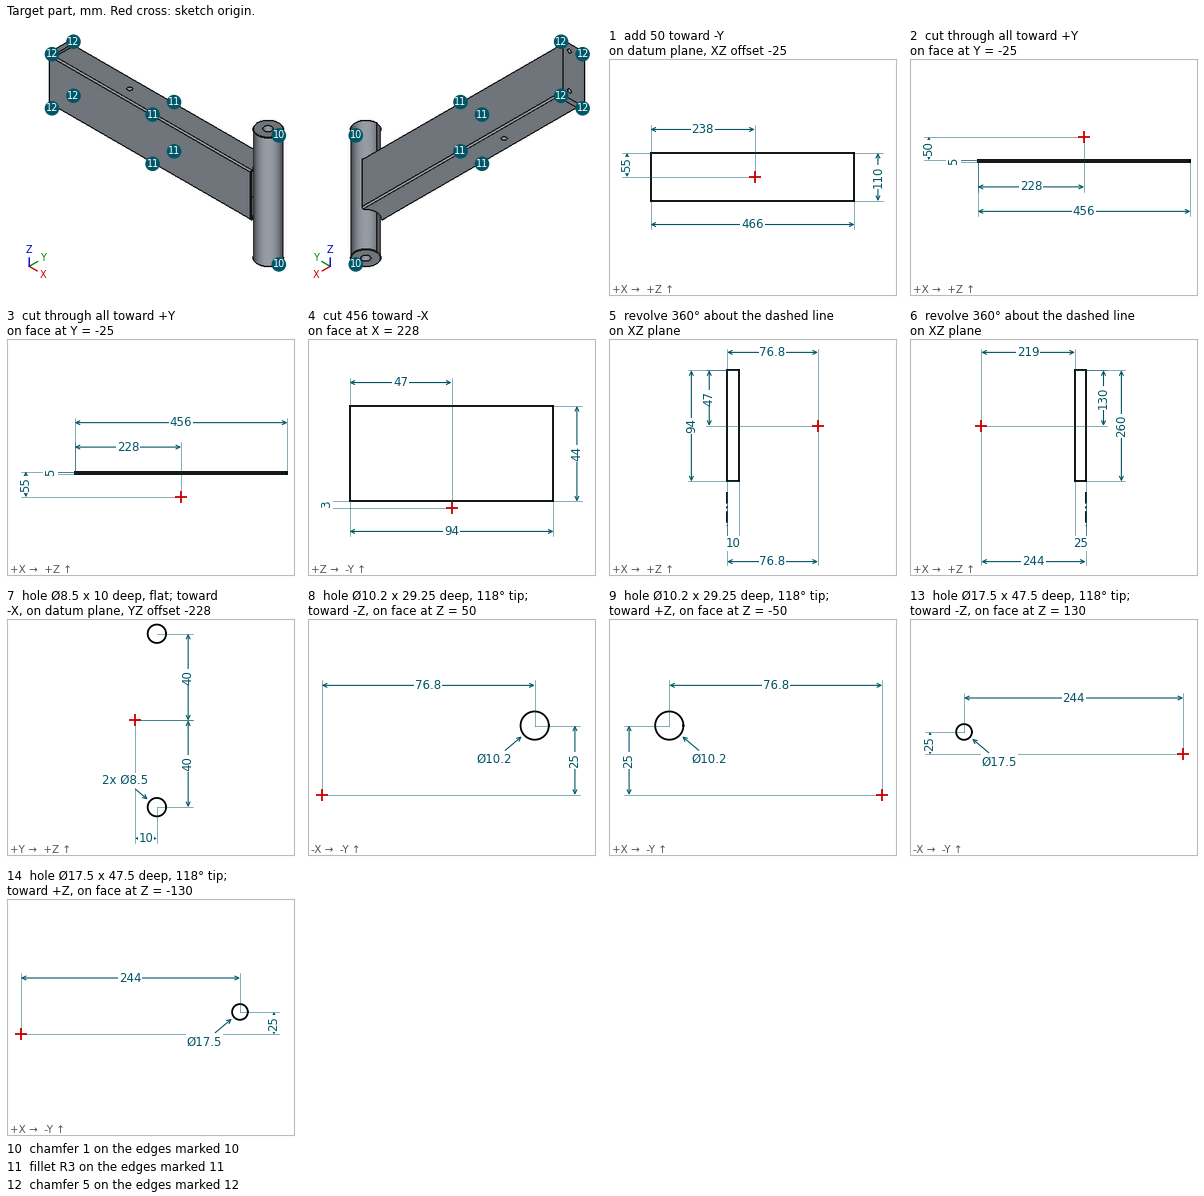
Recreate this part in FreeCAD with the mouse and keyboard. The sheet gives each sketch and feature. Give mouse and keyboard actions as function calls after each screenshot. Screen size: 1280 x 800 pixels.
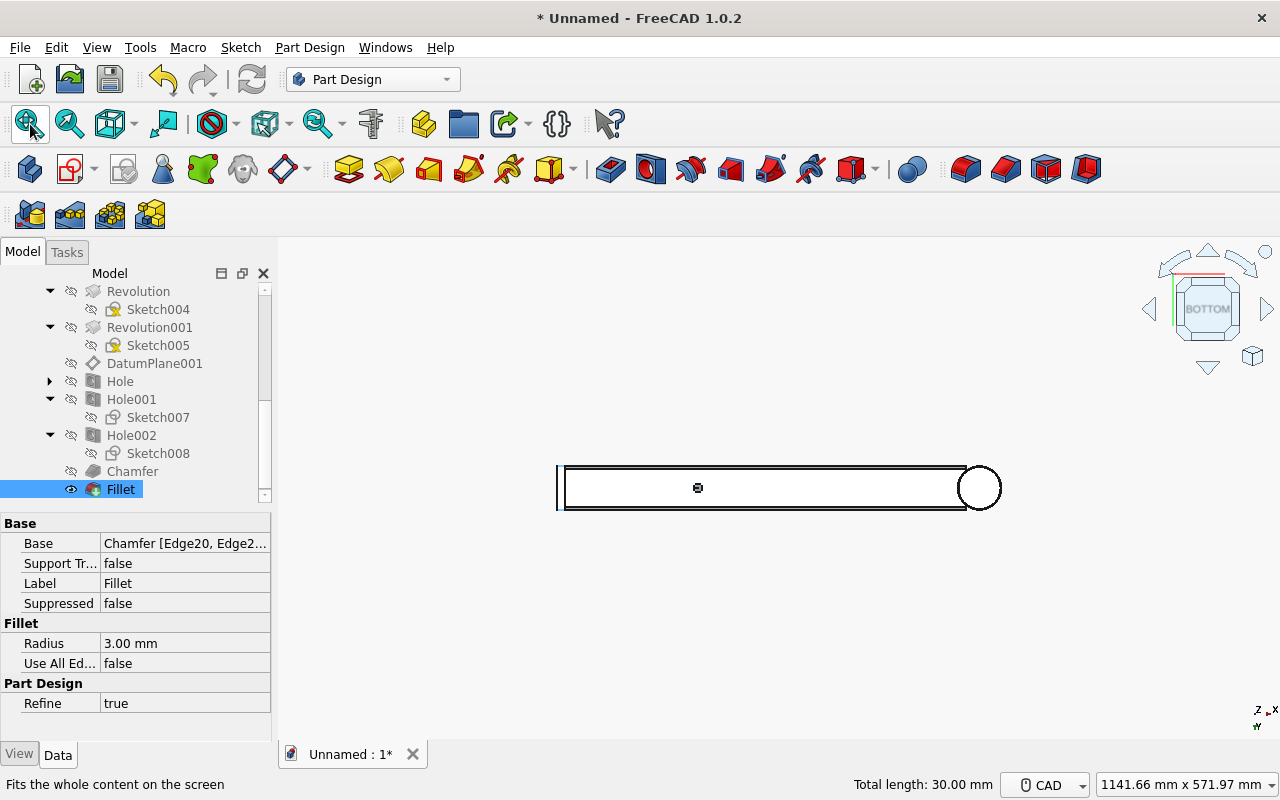
key(4)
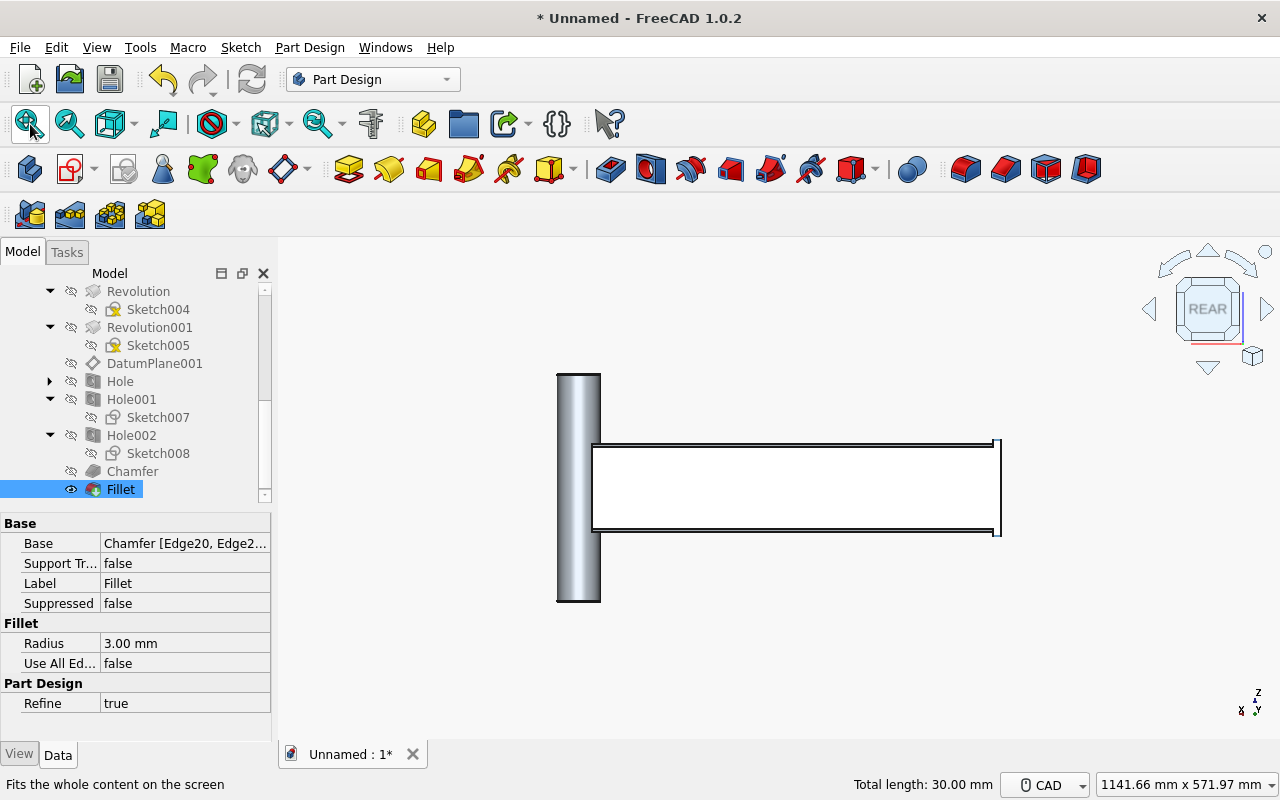
scroll(997, 439, up, 8)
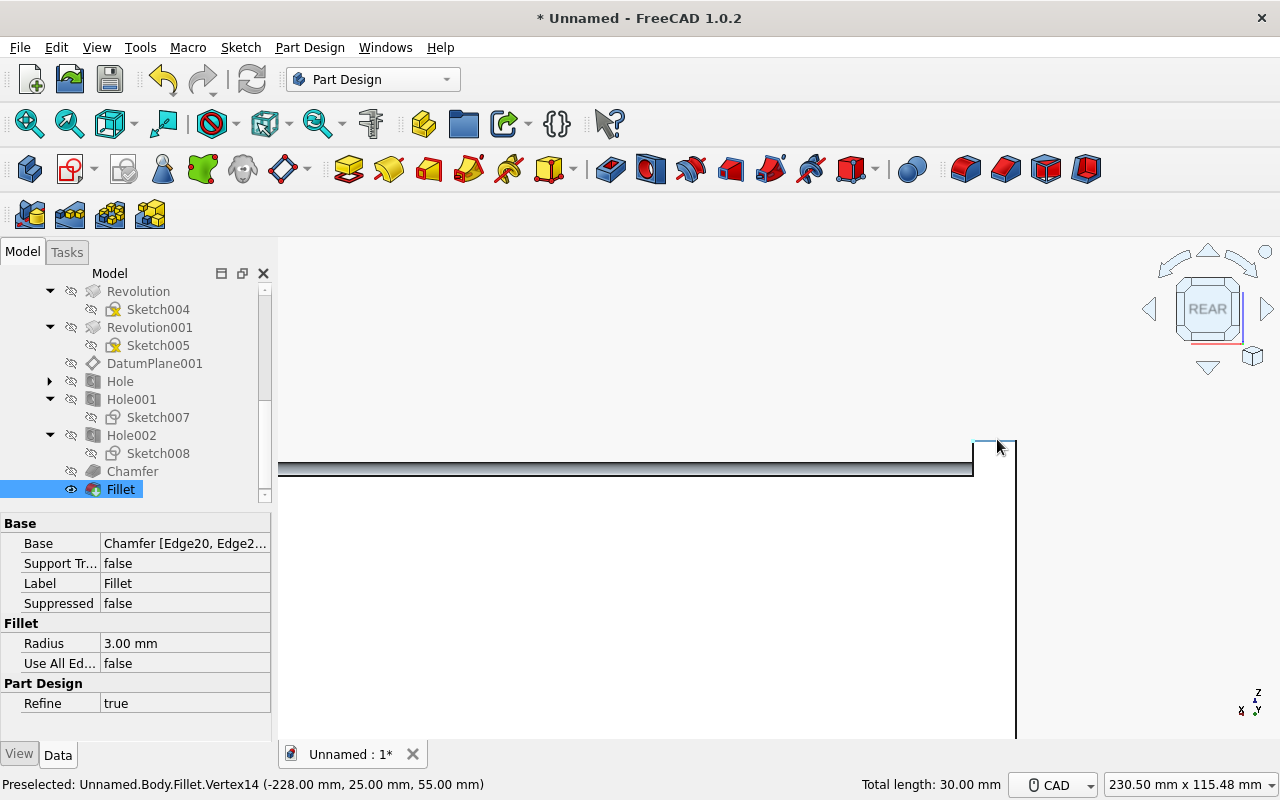
click(30, 124)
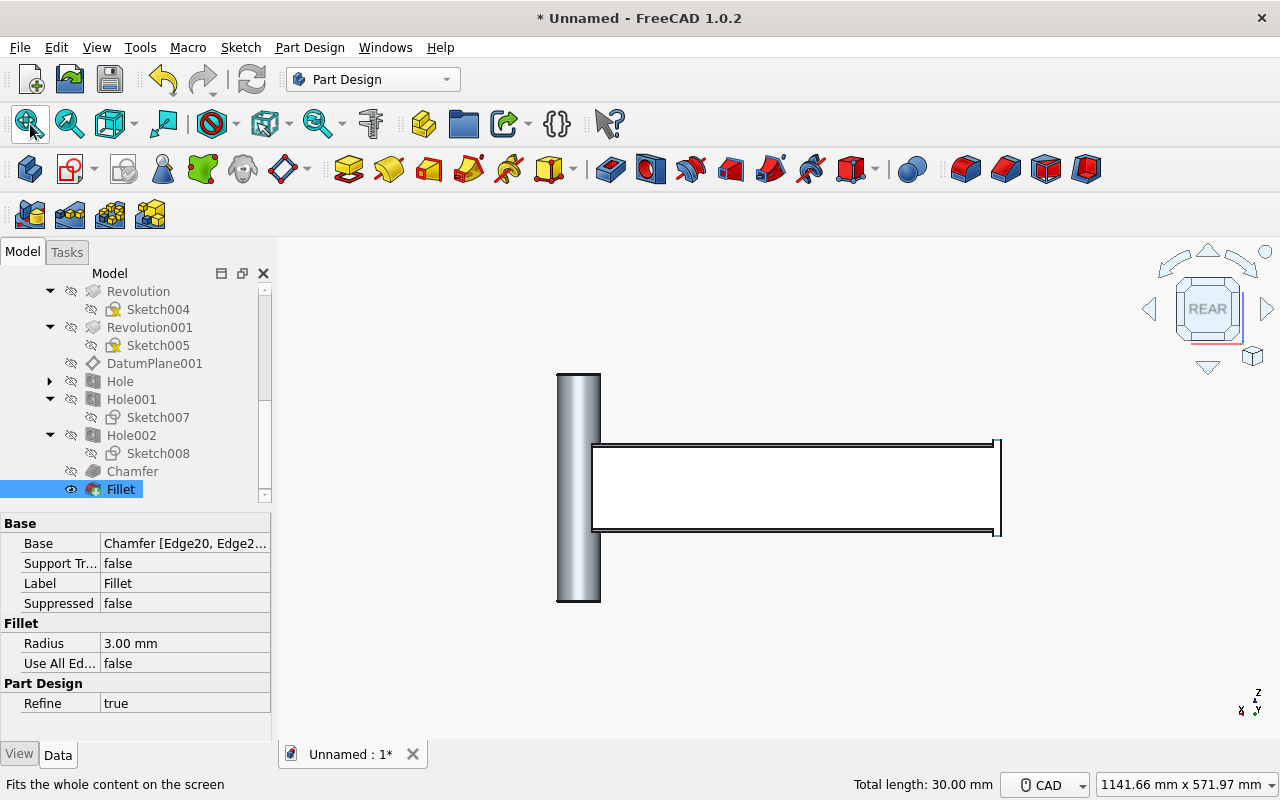
key(6)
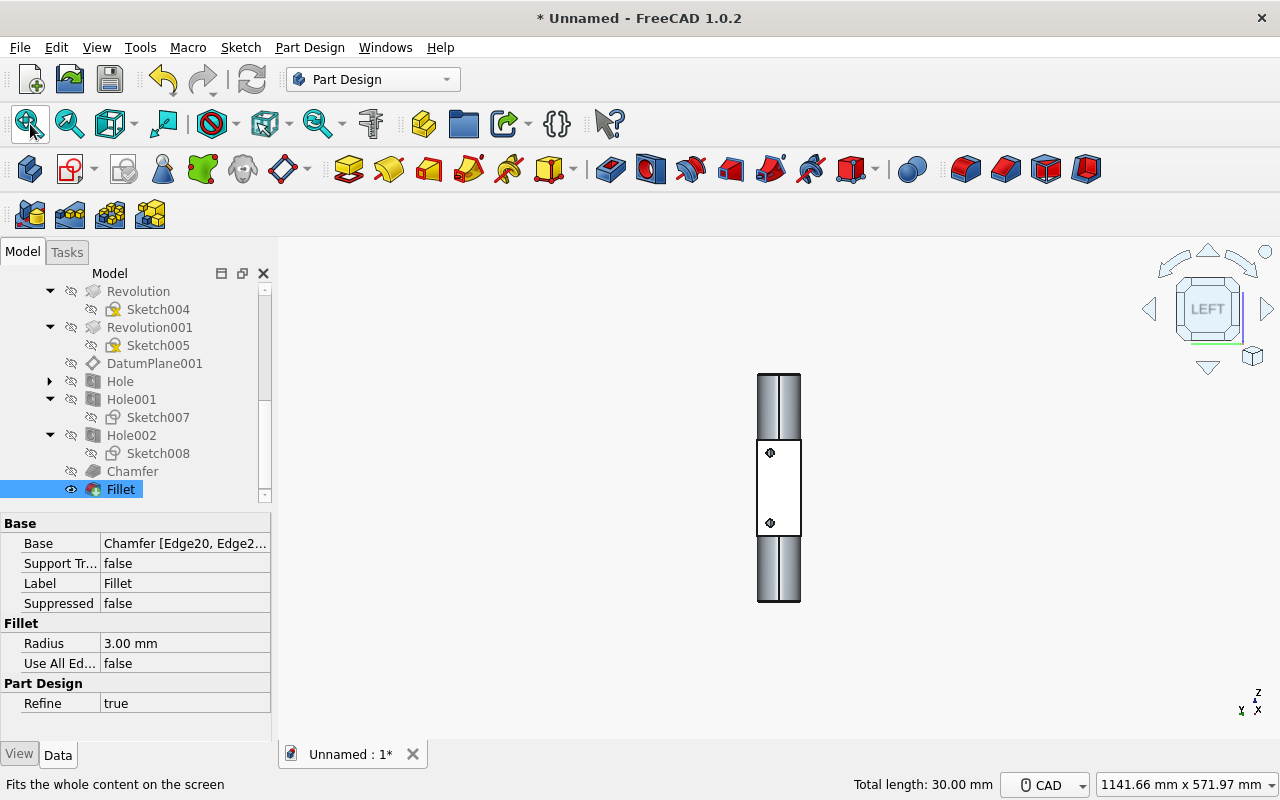
scroll(801, 439, up, 8)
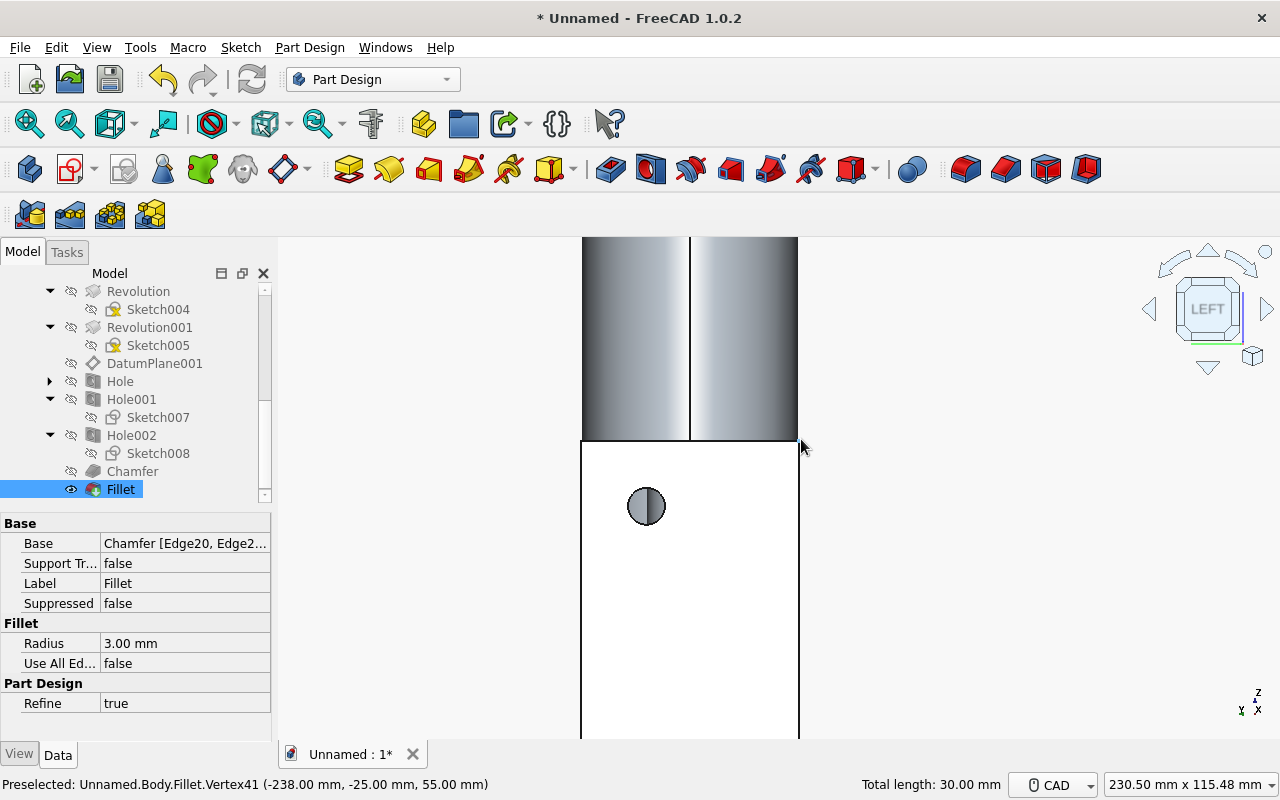
click(30, 124)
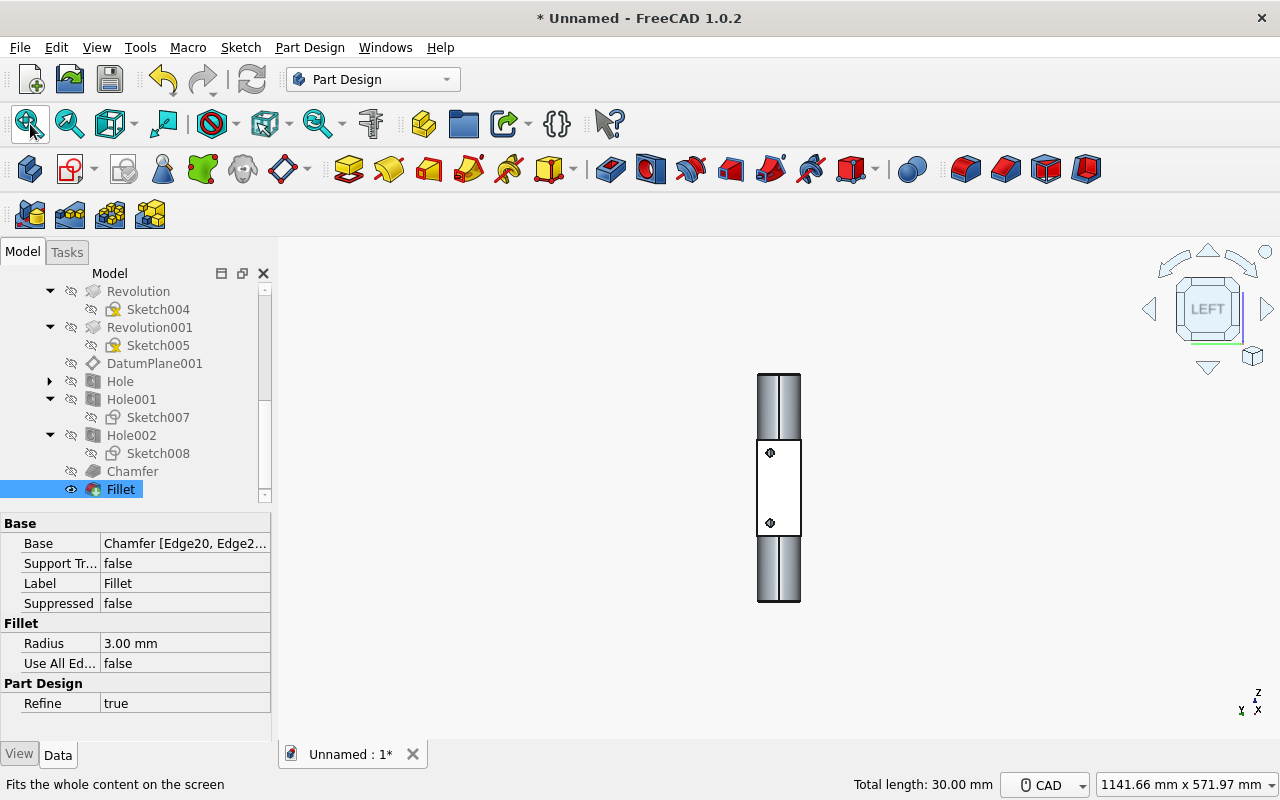
key(v)
key(3)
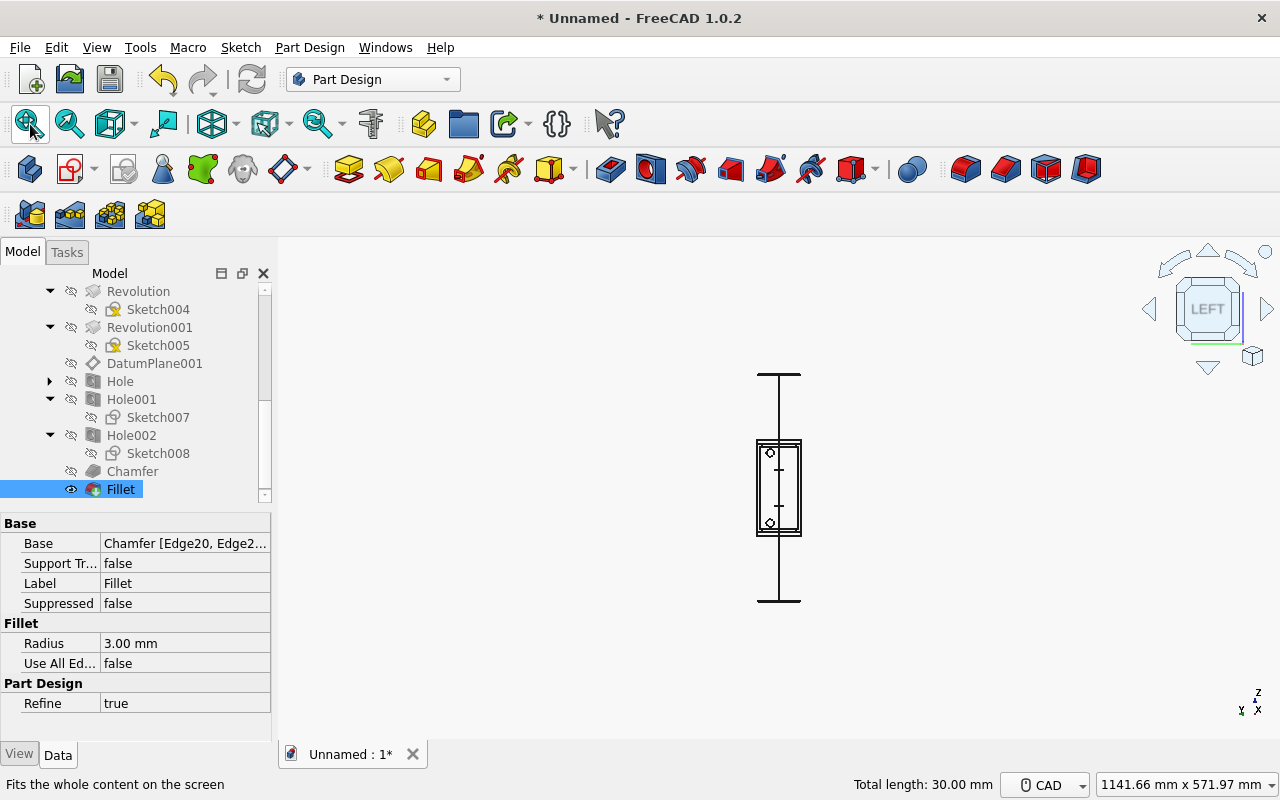
key(0)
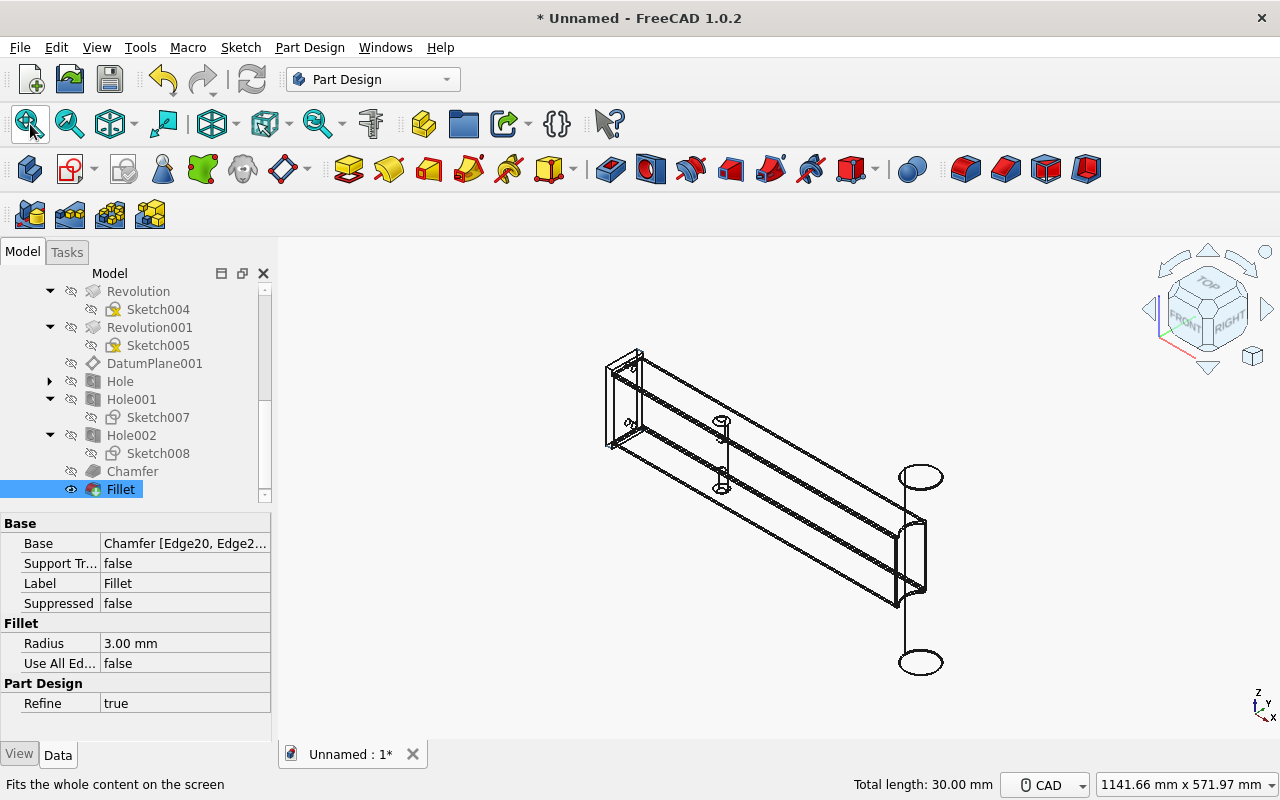
scroll(609, 368, up, 8)